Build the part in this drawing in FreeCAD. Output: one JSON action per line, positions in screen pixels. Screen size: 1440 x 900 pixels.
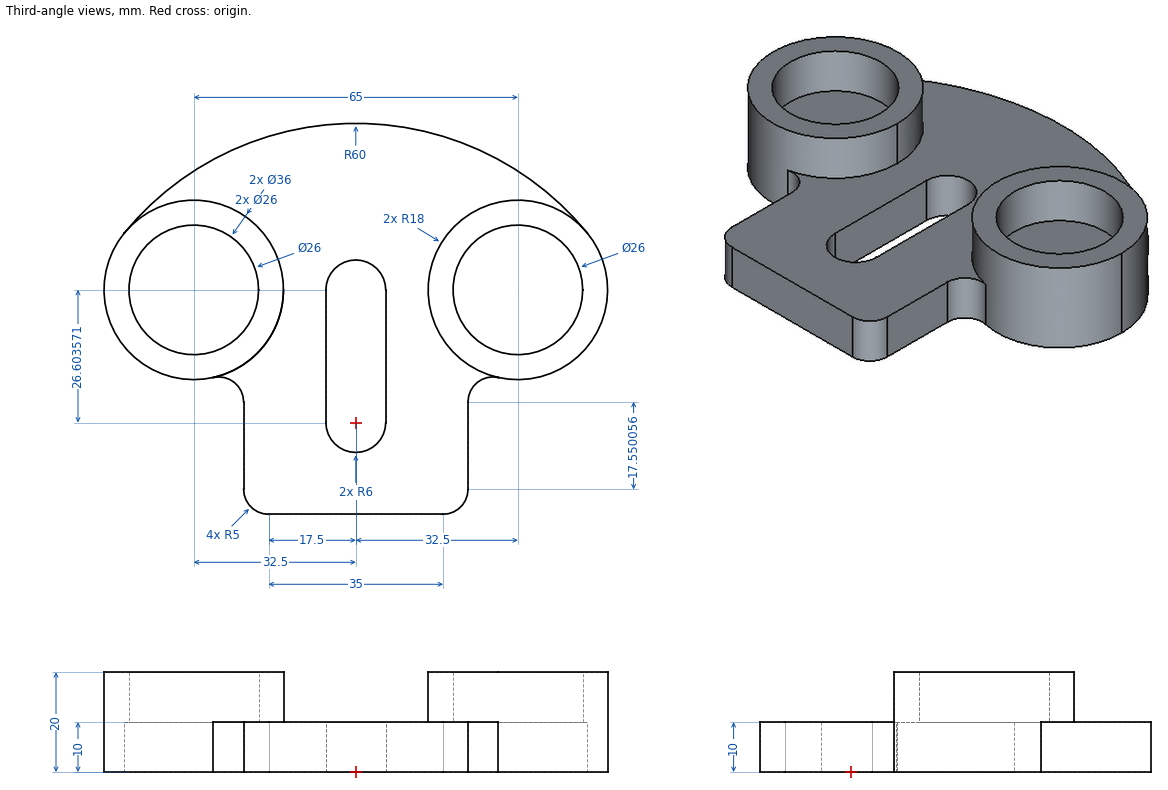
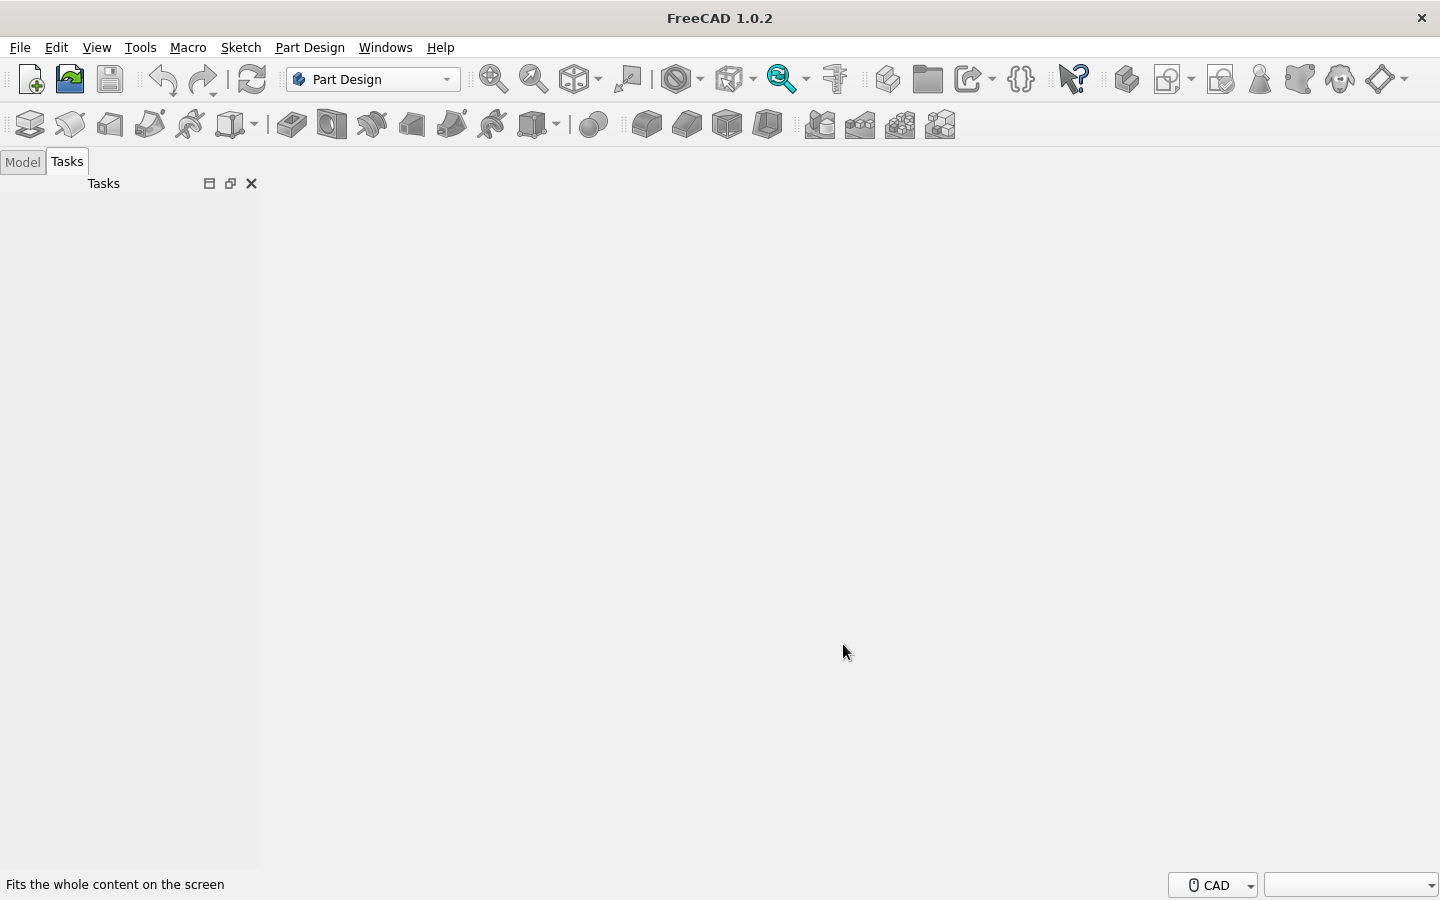
{"action": "left_click", "coordinate": [30, 80]}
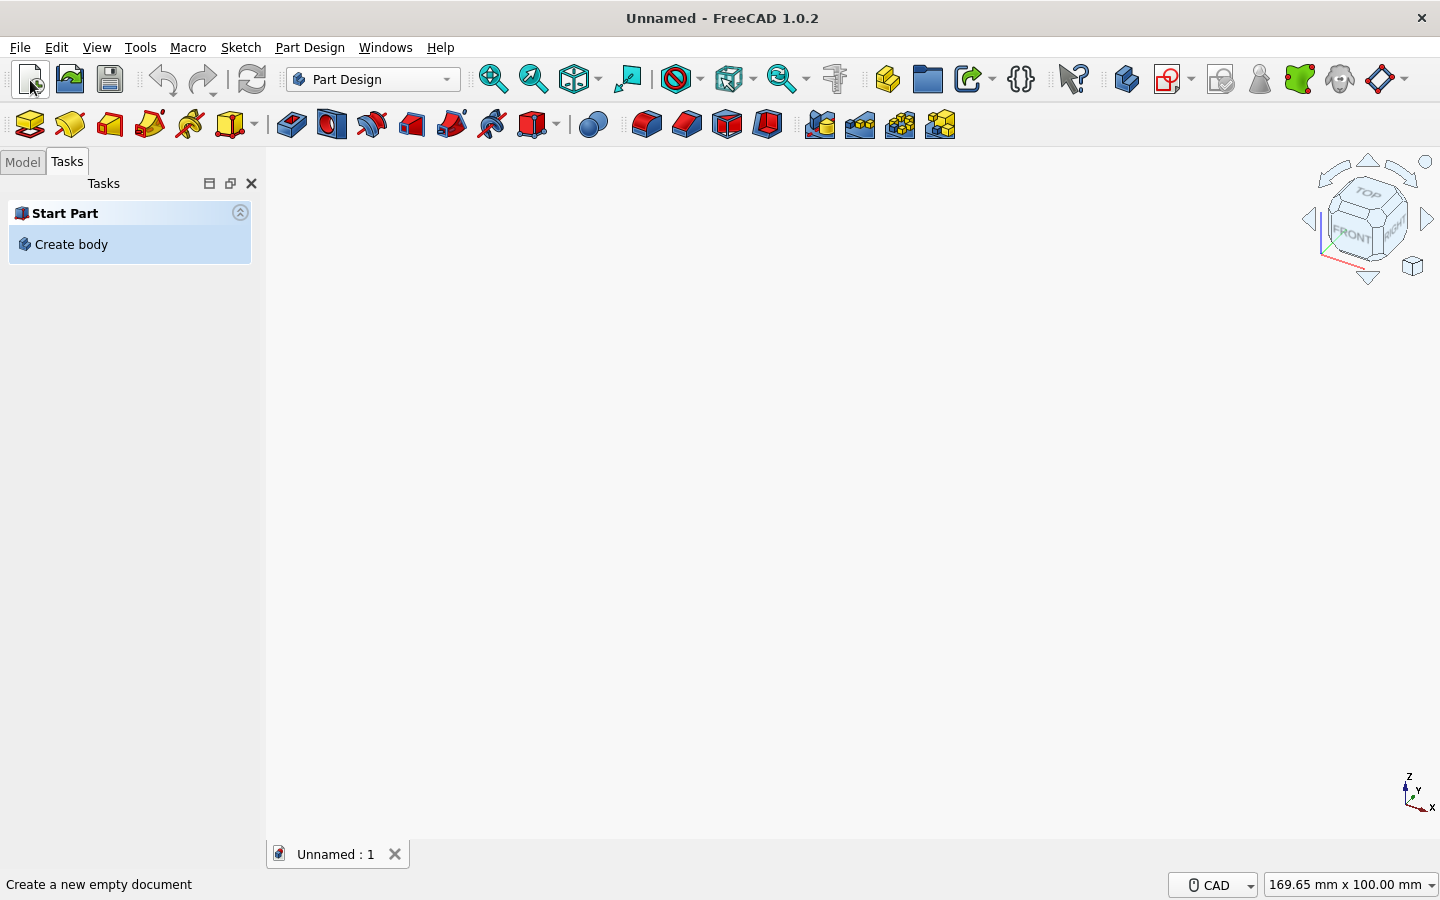
{"action": "left_click", "coordinate": [1168, 80]}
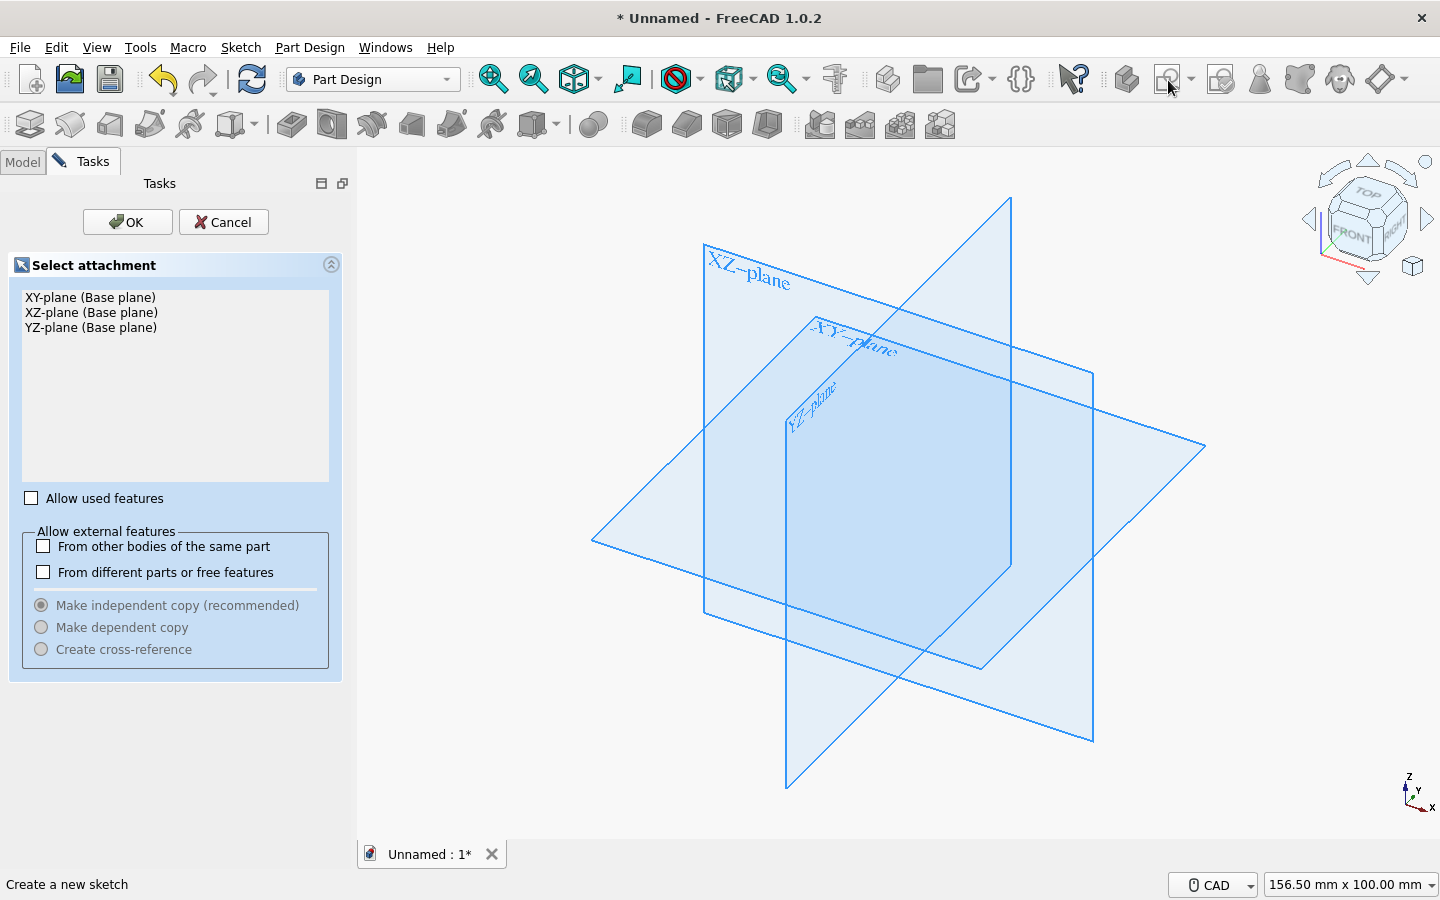
{"action": "left_click", "coordinate": [82, 298]}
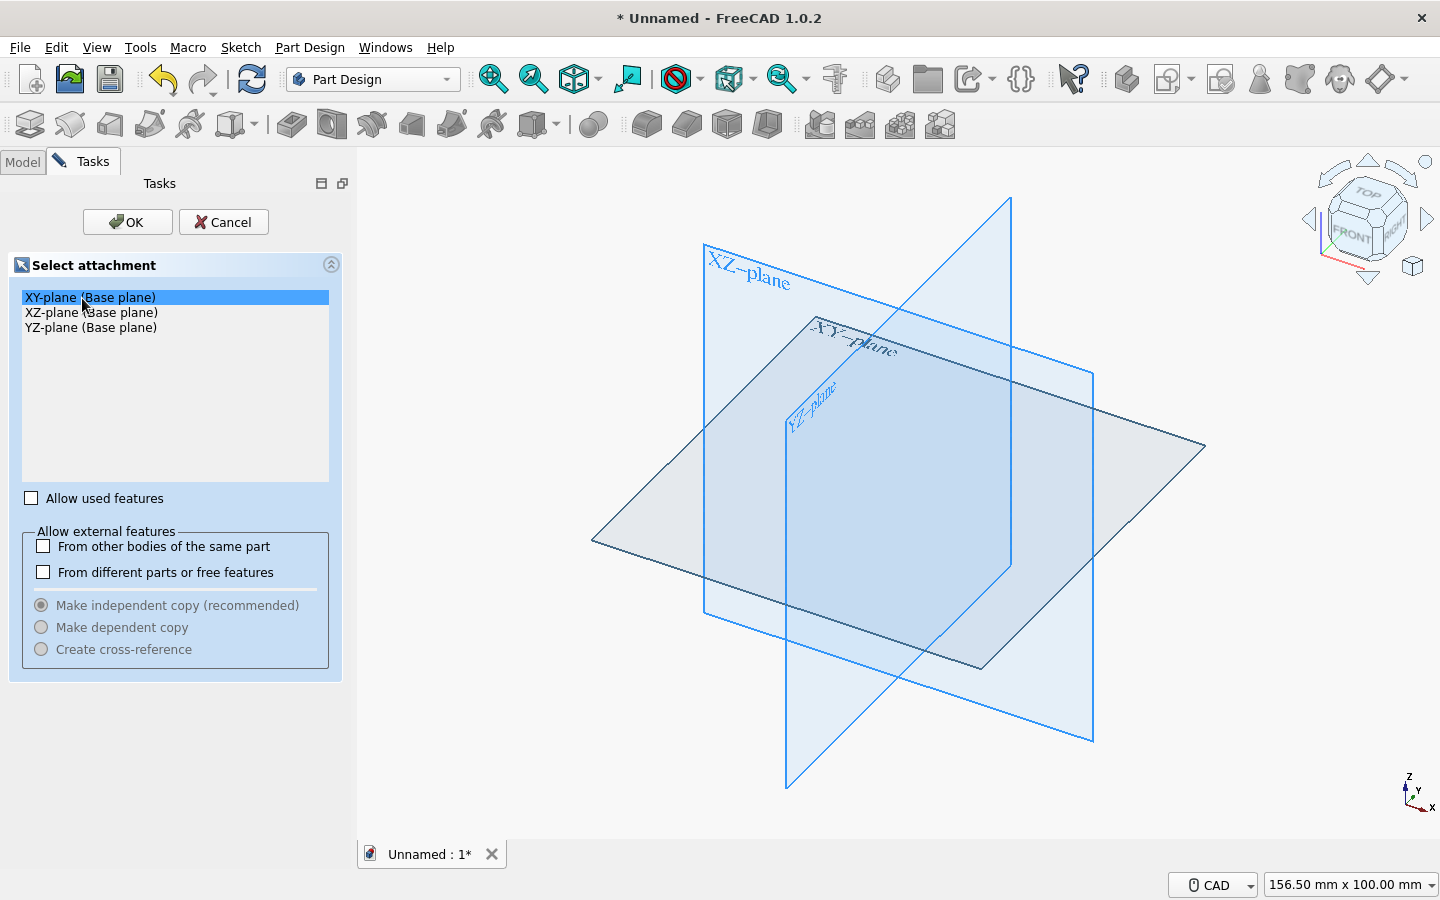
{"action": "left_click", "coordinate": [128, 222]}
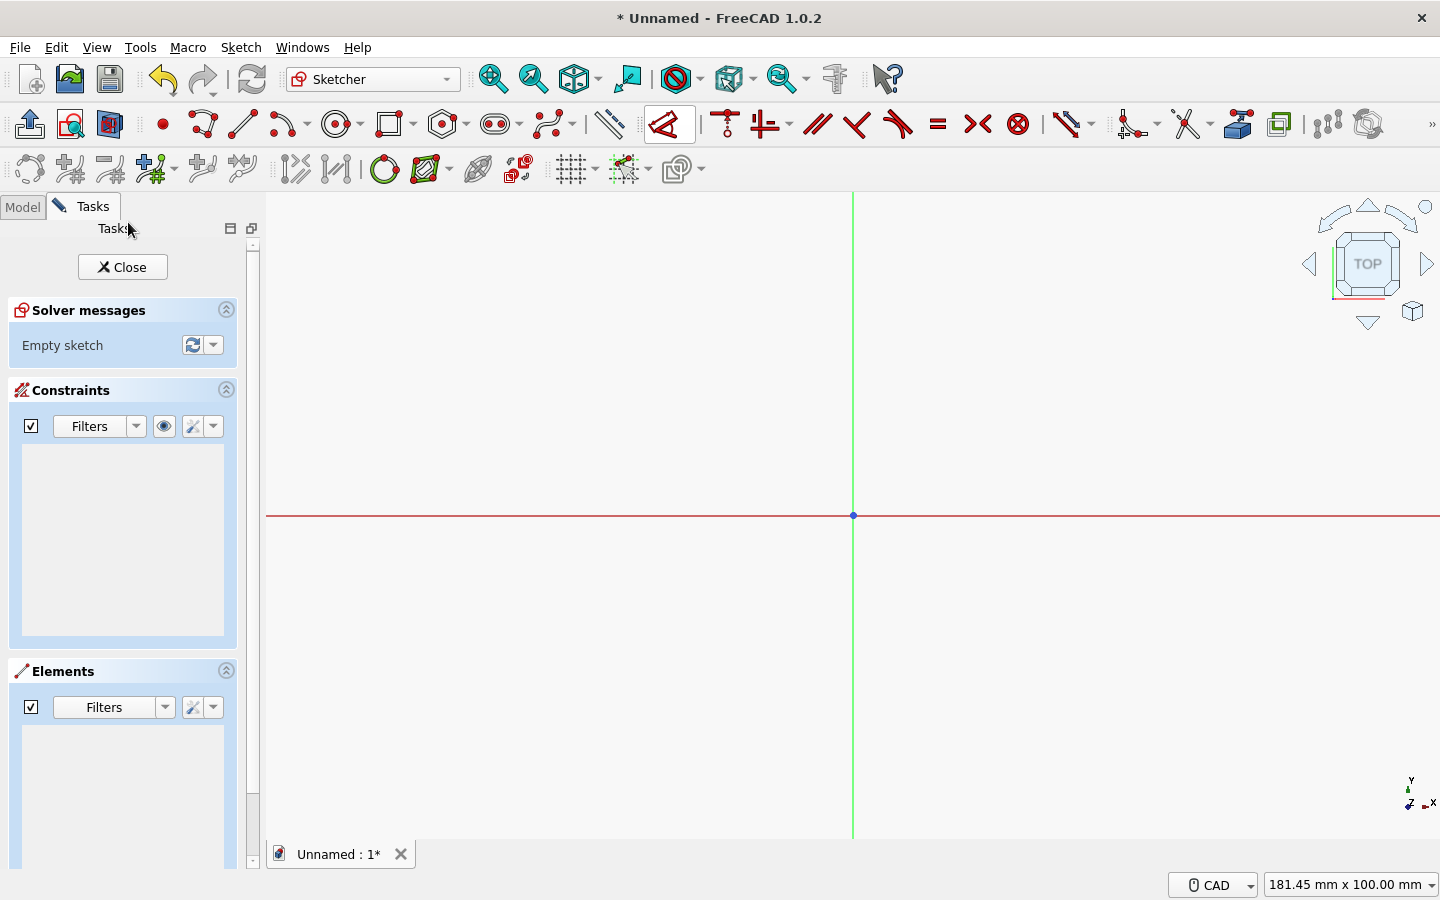
{"action": "scroll", "coordinate": [475, 811], "scroll_direction": "down", "scroll_amount": 1}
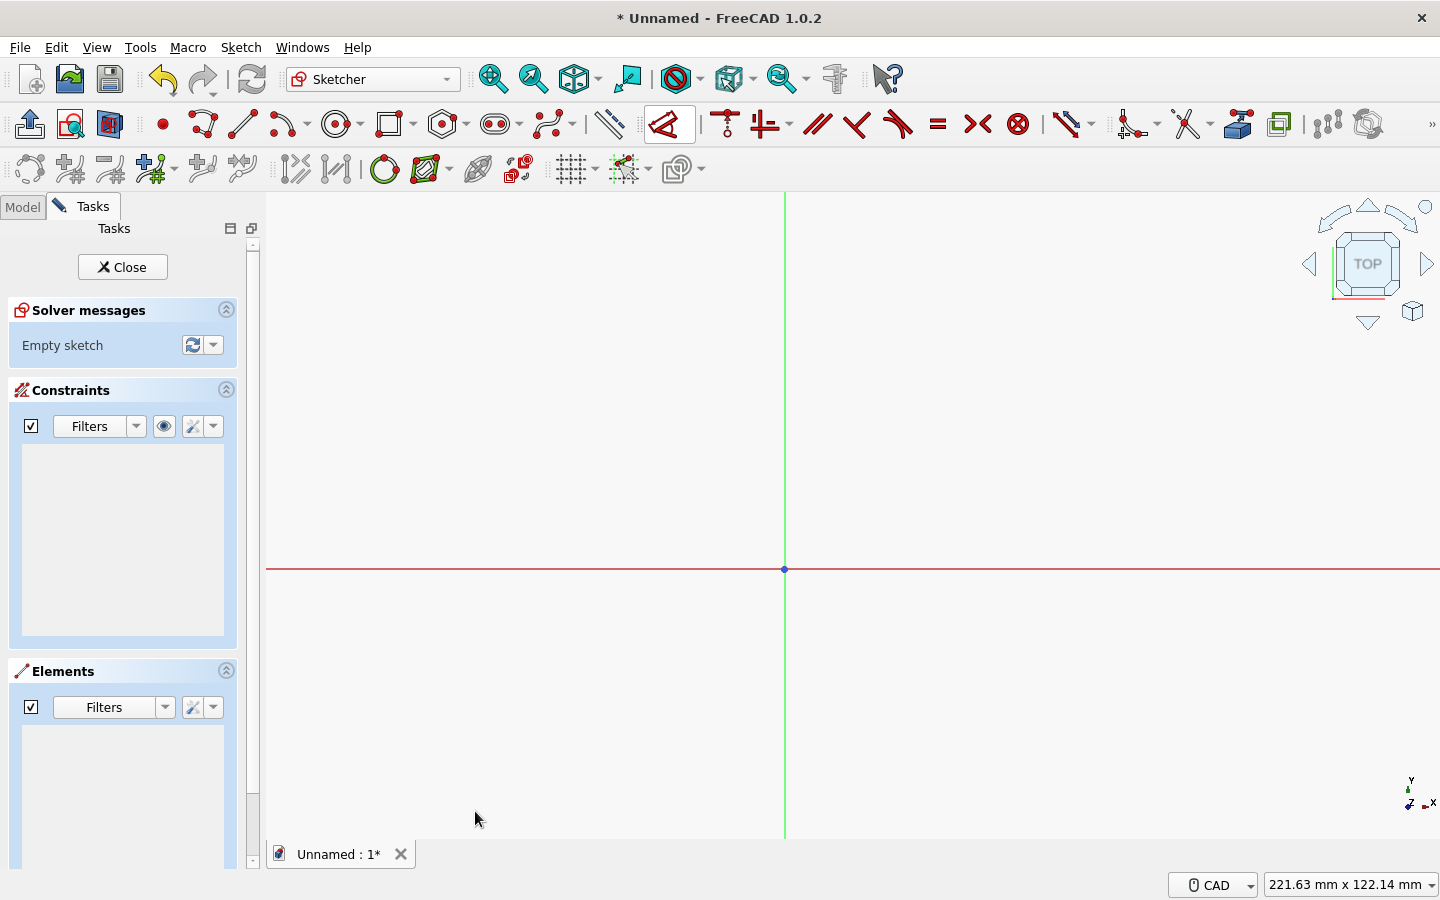
{"action": "key", "text": "g l"}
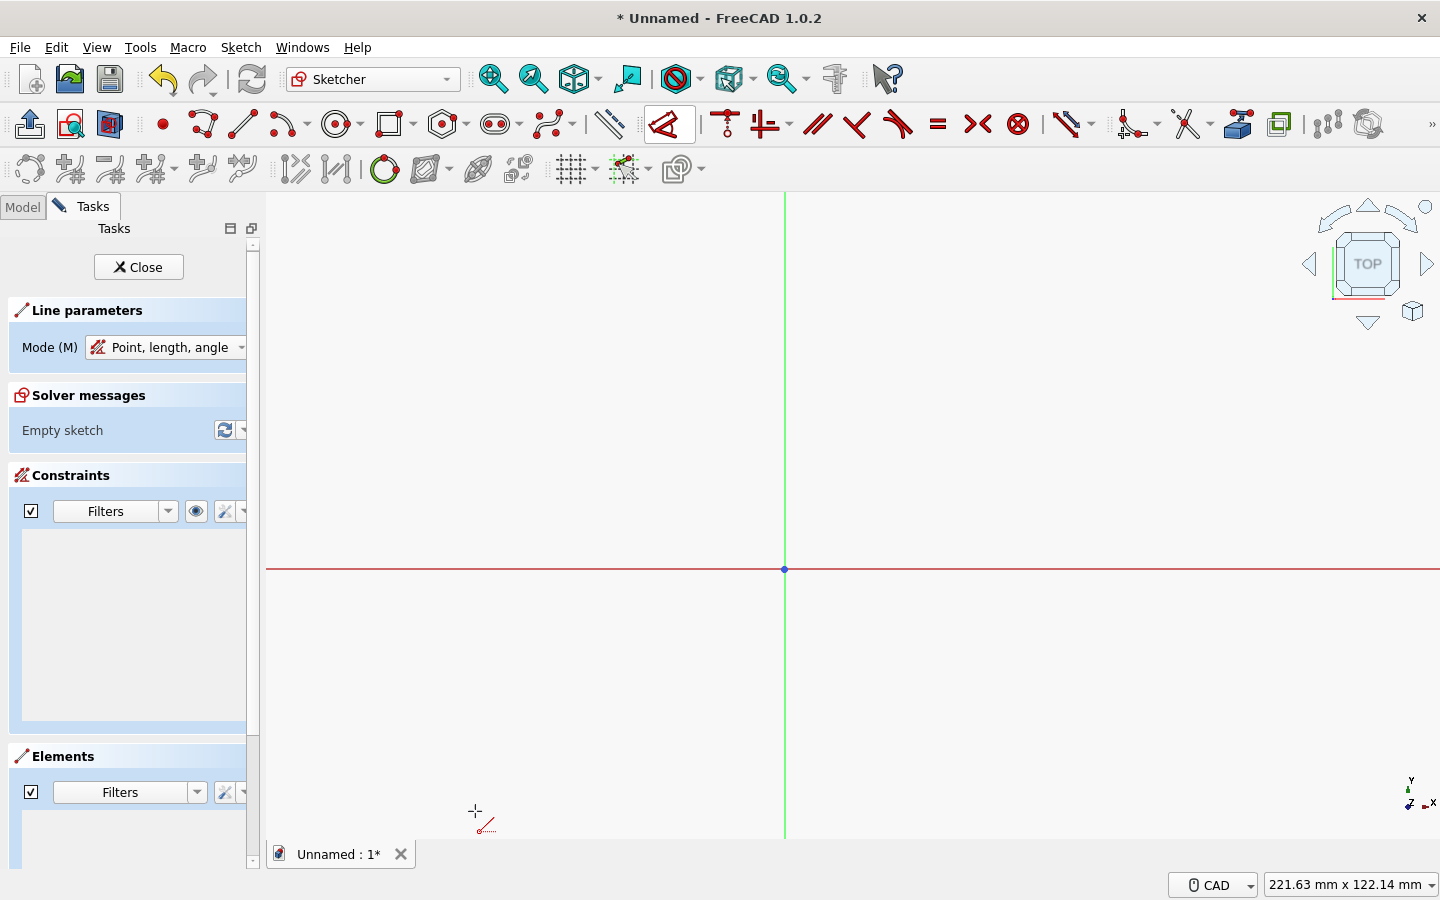
{"action": "left_click", "coordinate": [692, 667]}
{"action": "left_click", "coordinate": [877, 667]}